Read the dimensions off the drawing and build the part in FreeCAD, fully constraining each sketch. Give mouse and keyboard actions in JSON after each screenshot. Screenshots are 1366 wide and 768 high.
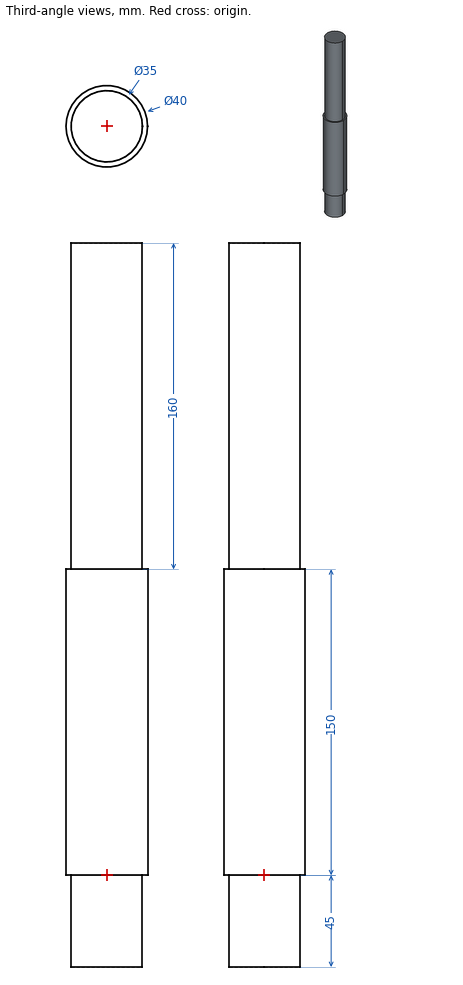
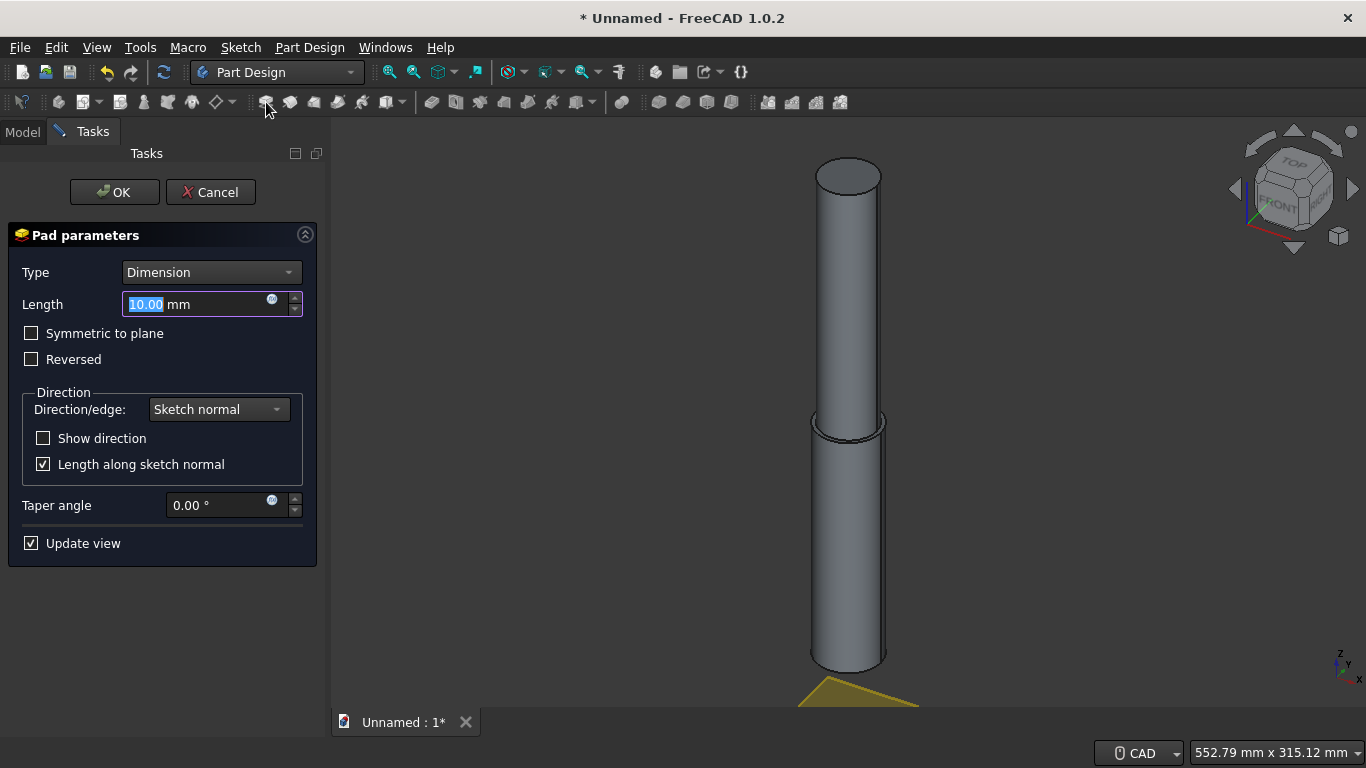
{"action": "type", "text": "45"}
{"action": "key", "text": "Tab"}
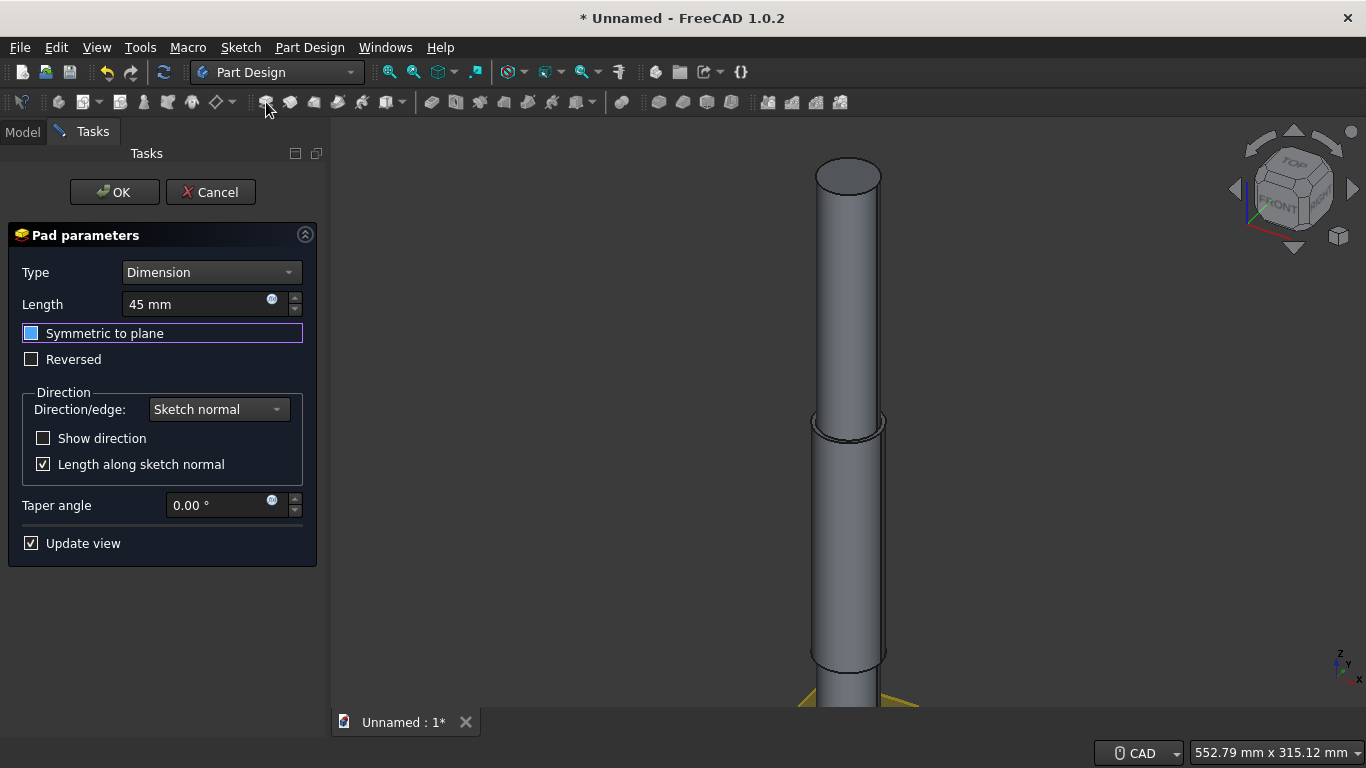
{"action": "left_click", "coordinate": [115, 192]}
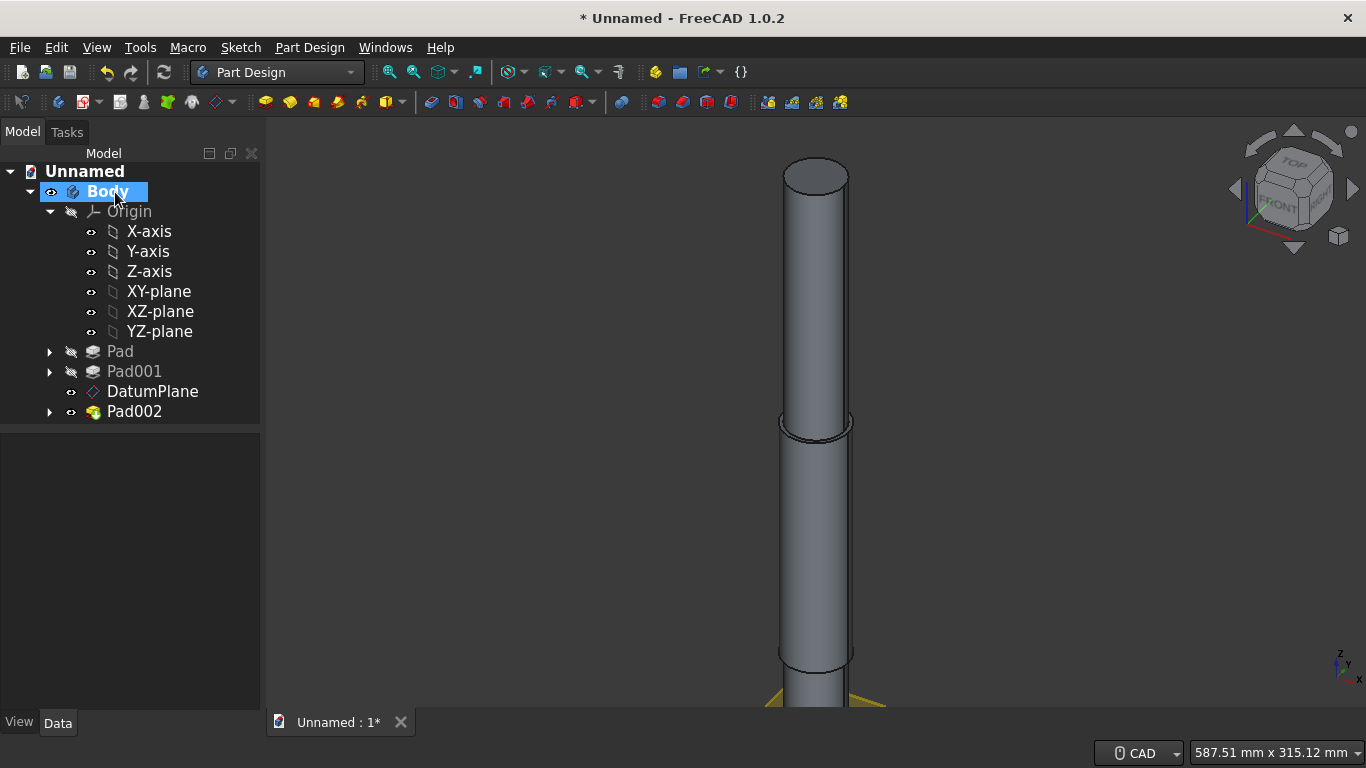
{"action": "left_click", "coordinate": [116, 392]}
{"action": "key", "text": "space"}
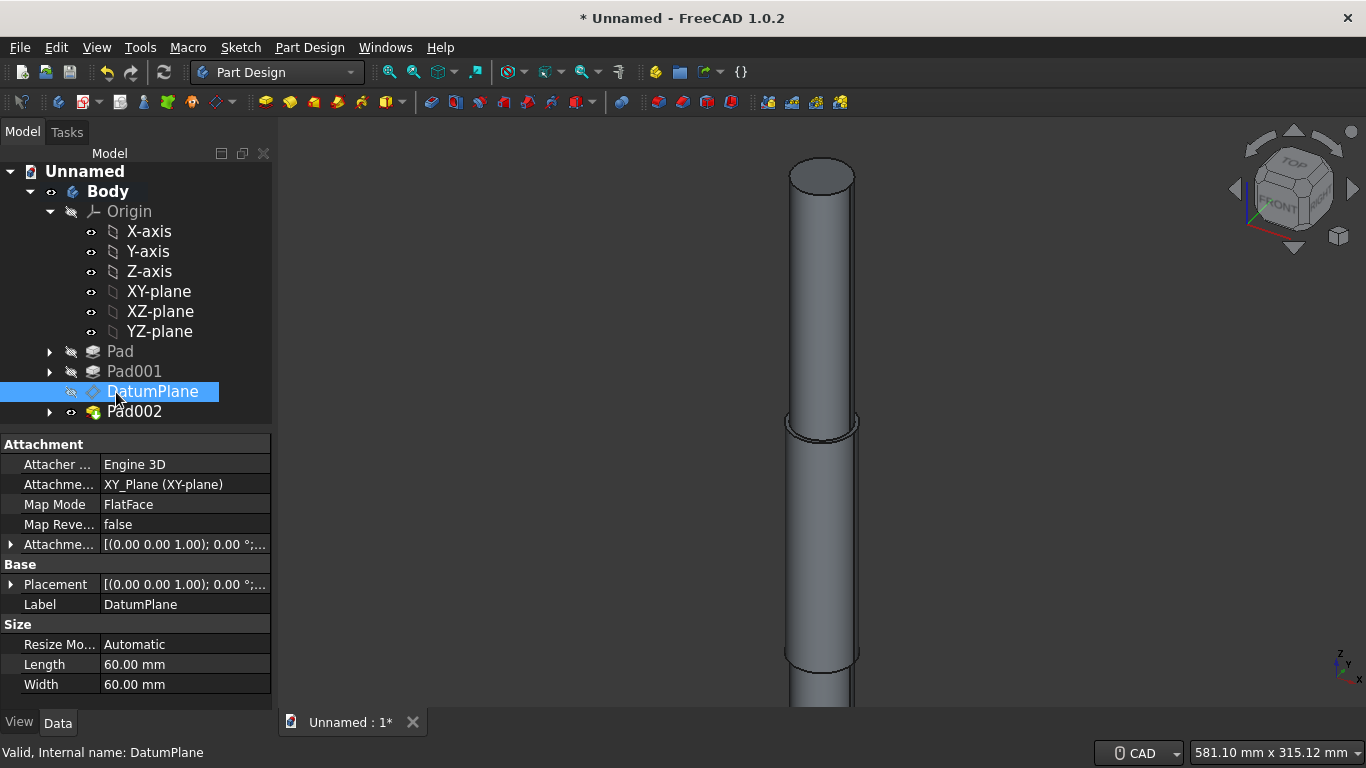
{"action": "key", "text": "0"}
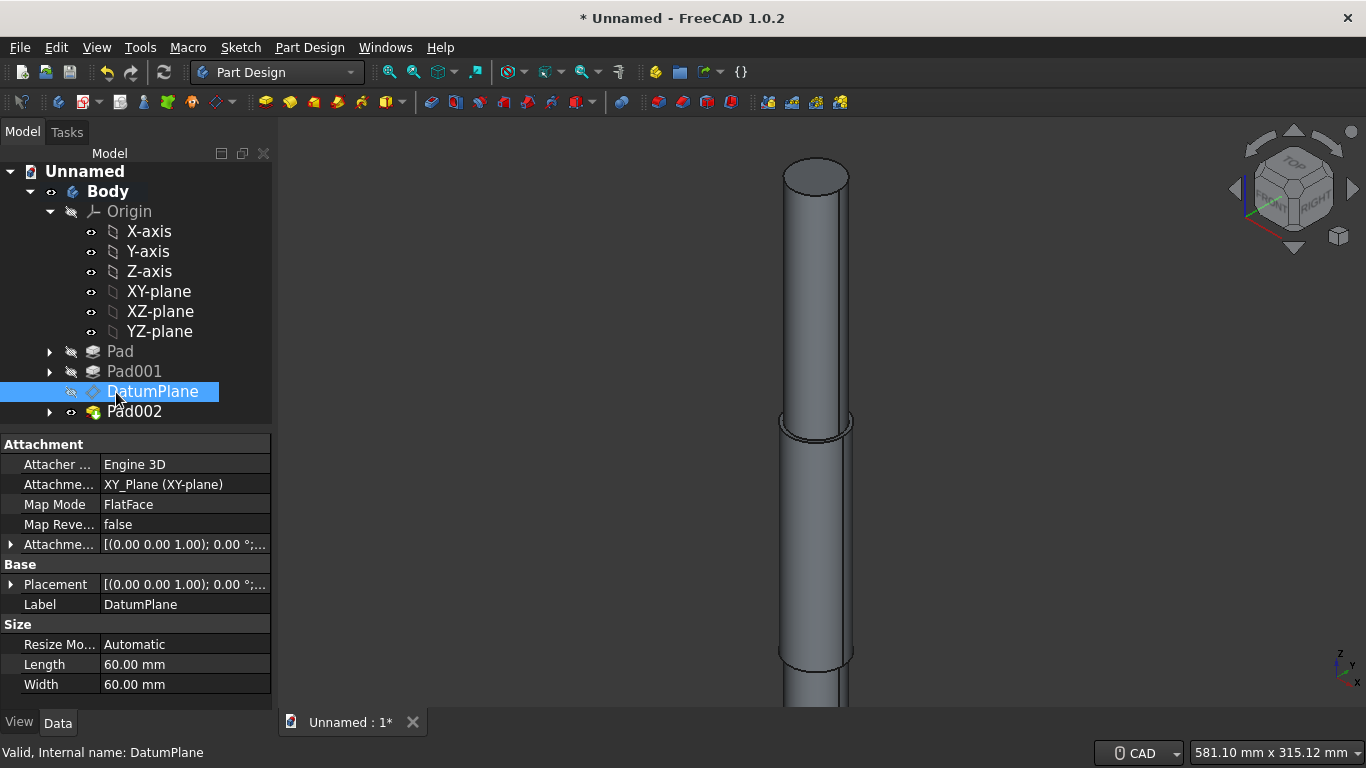
{"action": "key", "text": "v f"}